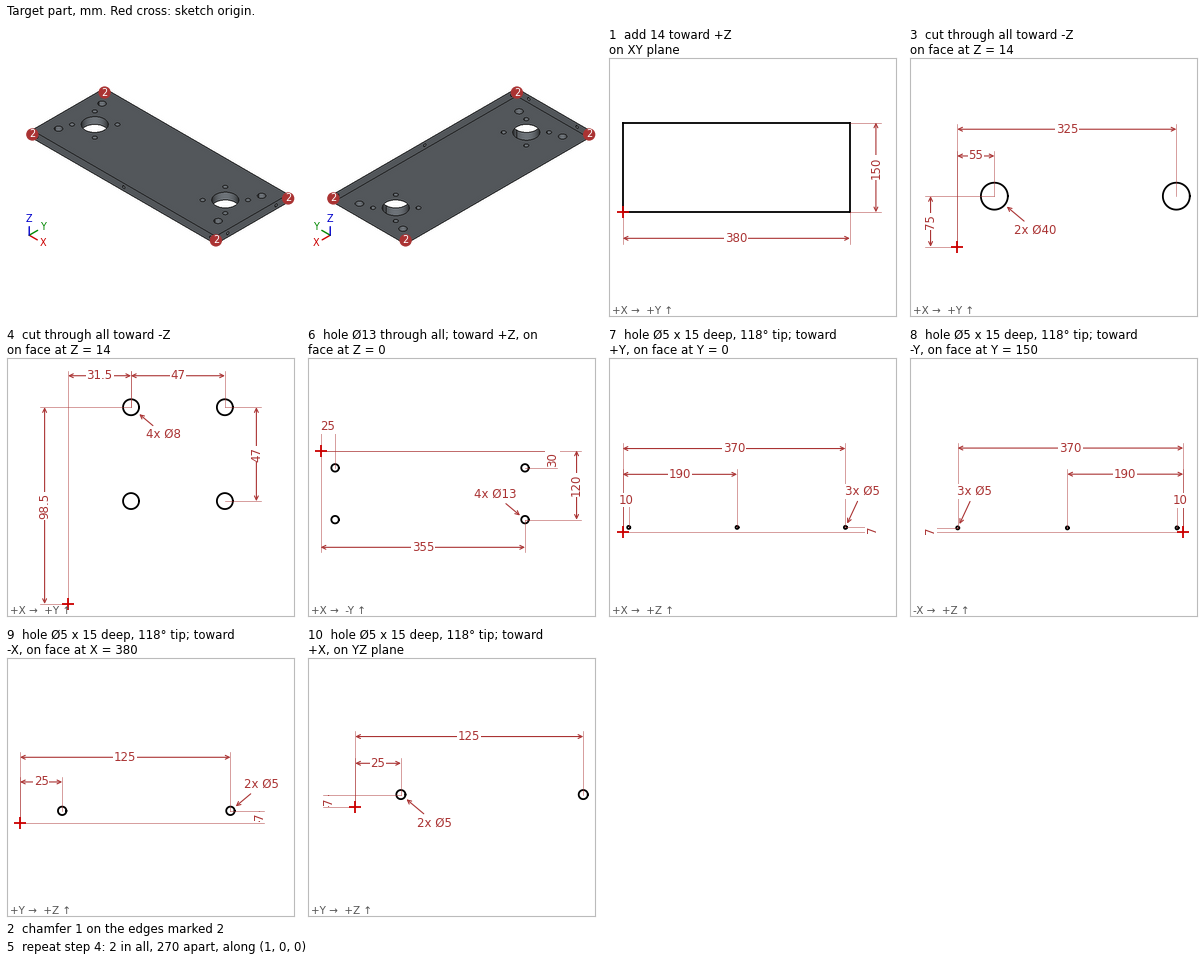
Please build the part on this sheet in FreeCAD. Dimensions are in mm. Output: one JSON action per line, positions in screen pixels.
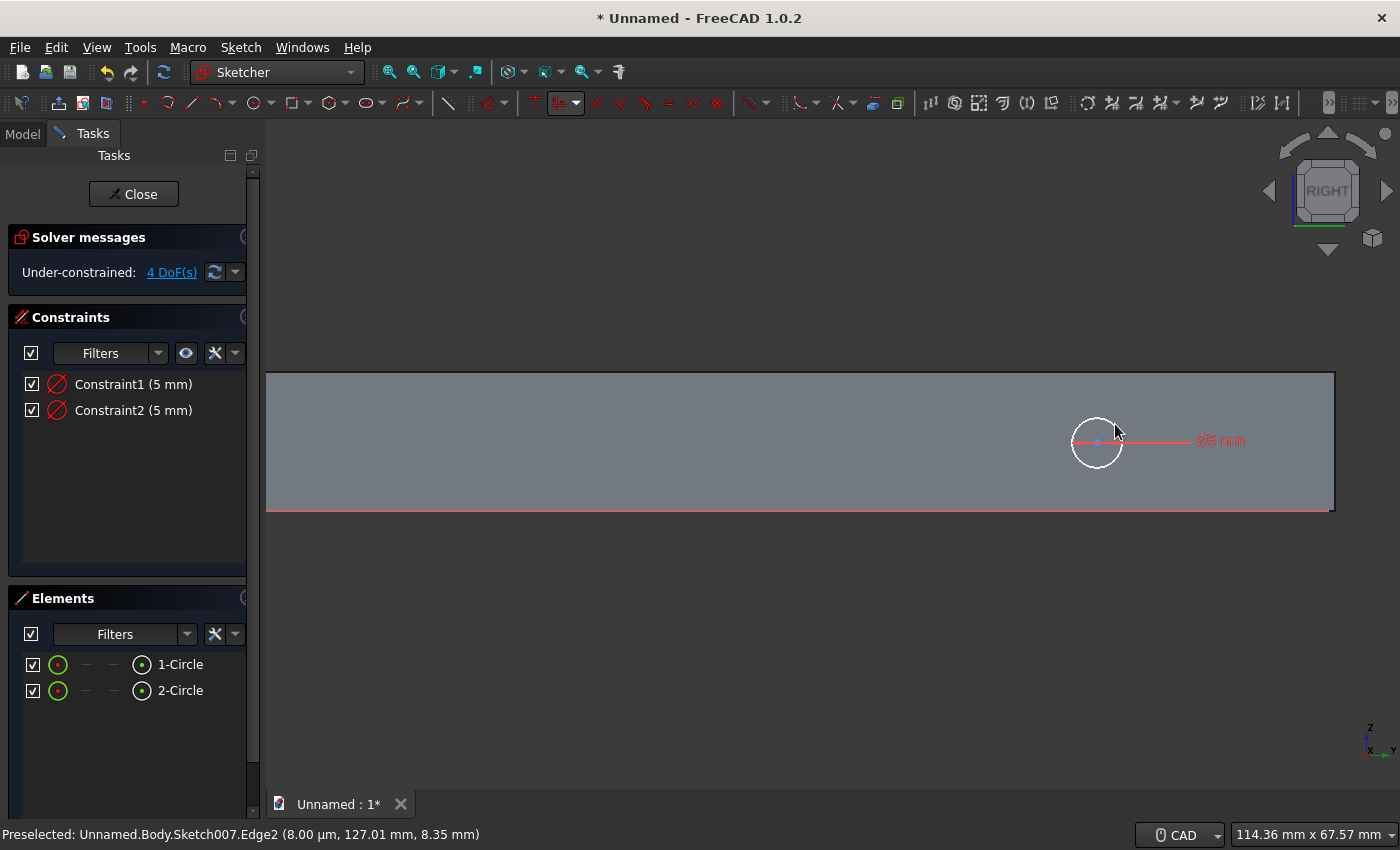
{"action": "scroll", "coordinate": [1099, 442], "scroll_direction": "down", "scroll_amount": 3}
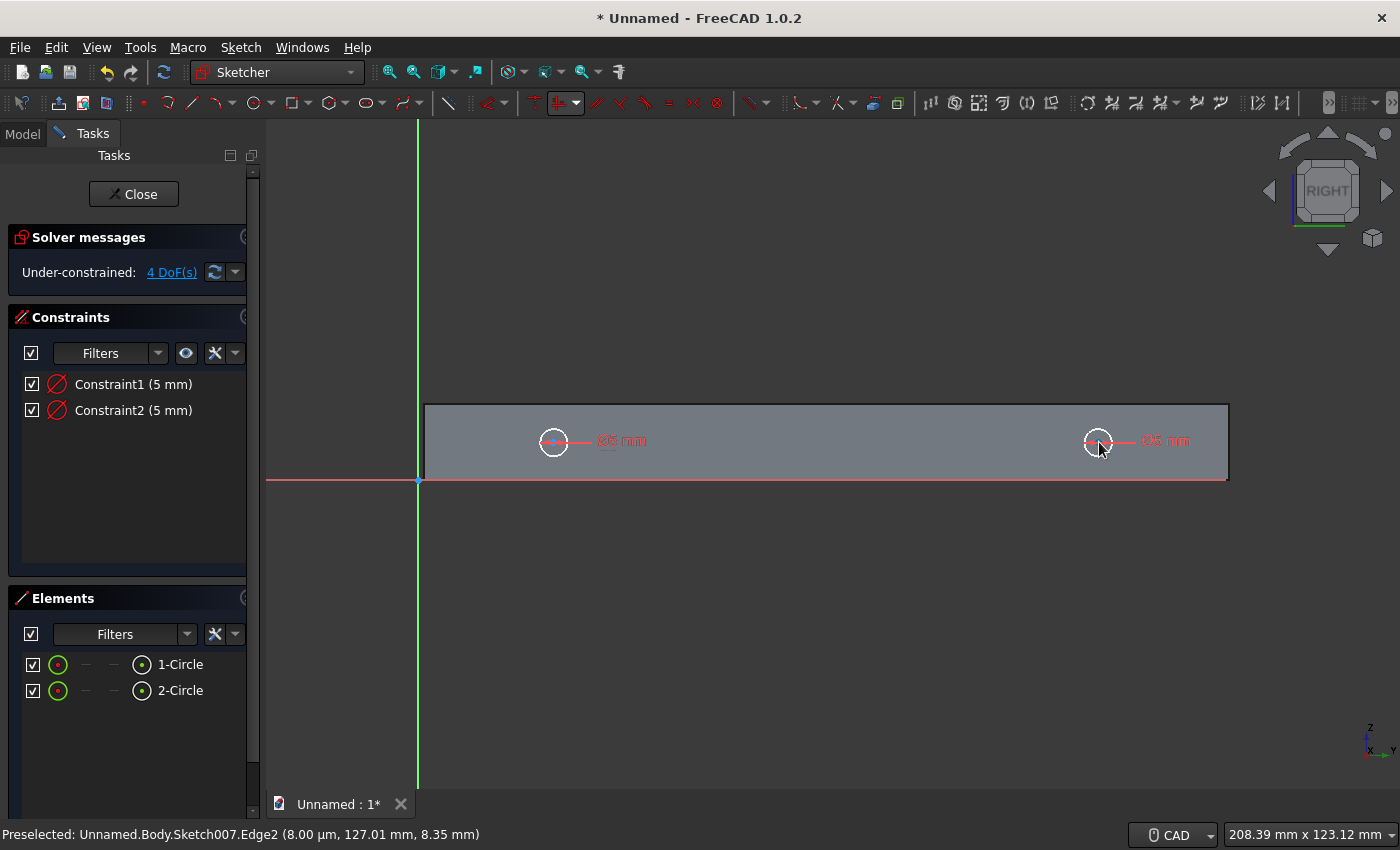
{"action": "left_click", "coordinate": [554, 443]}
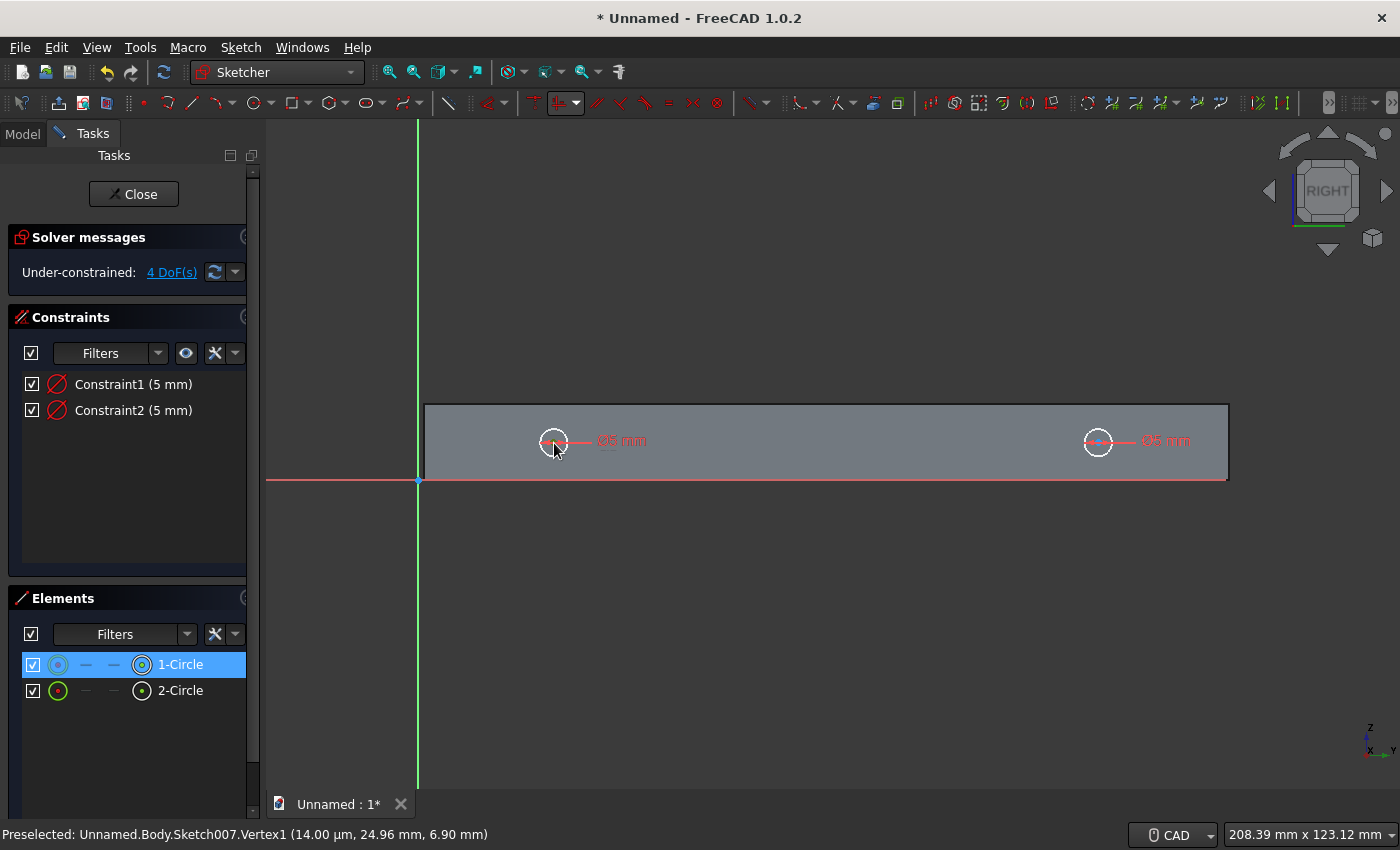
{"action": "left_click", "coordinate": [1098, 443]}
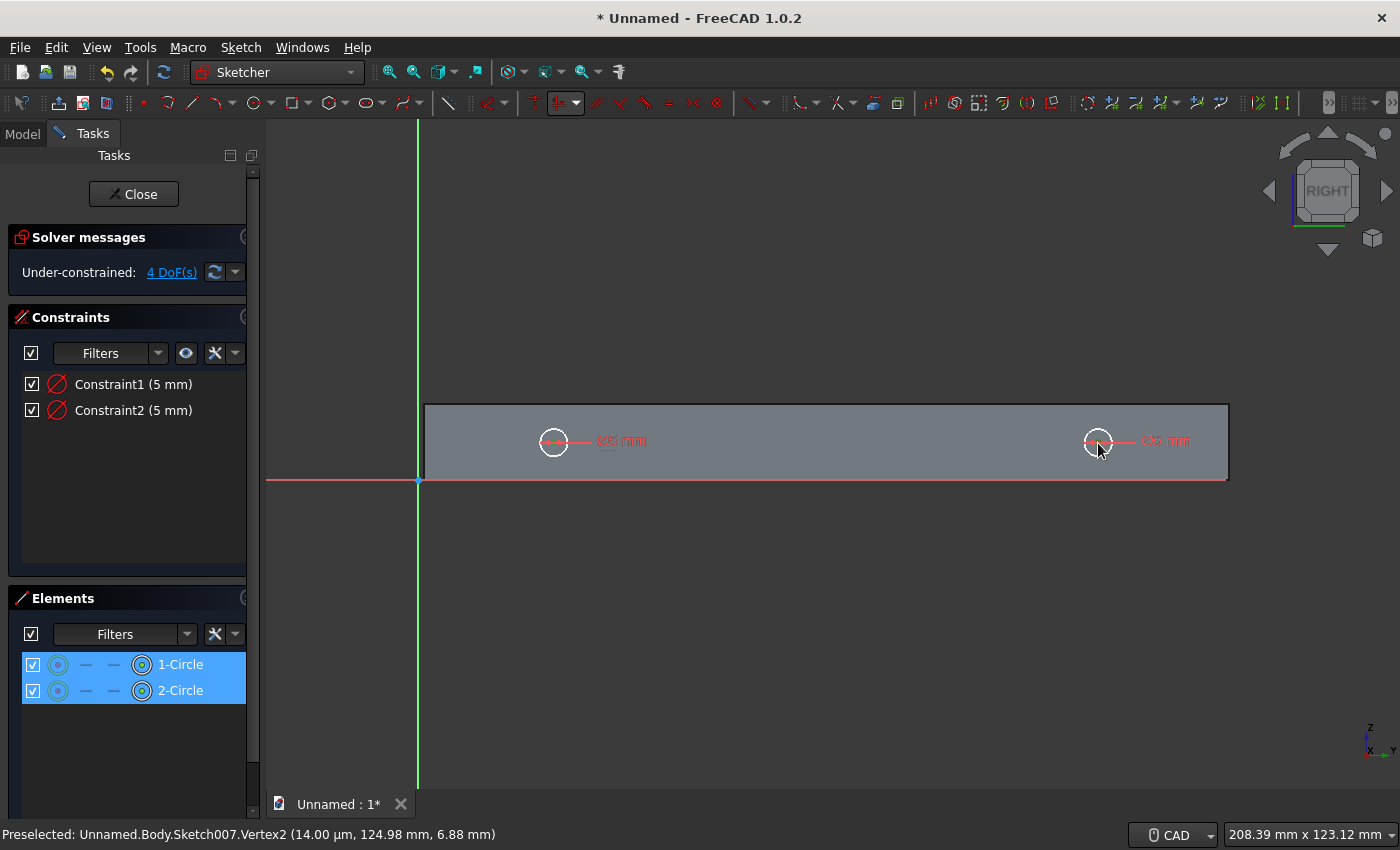
{"action": "key", "text": "h"}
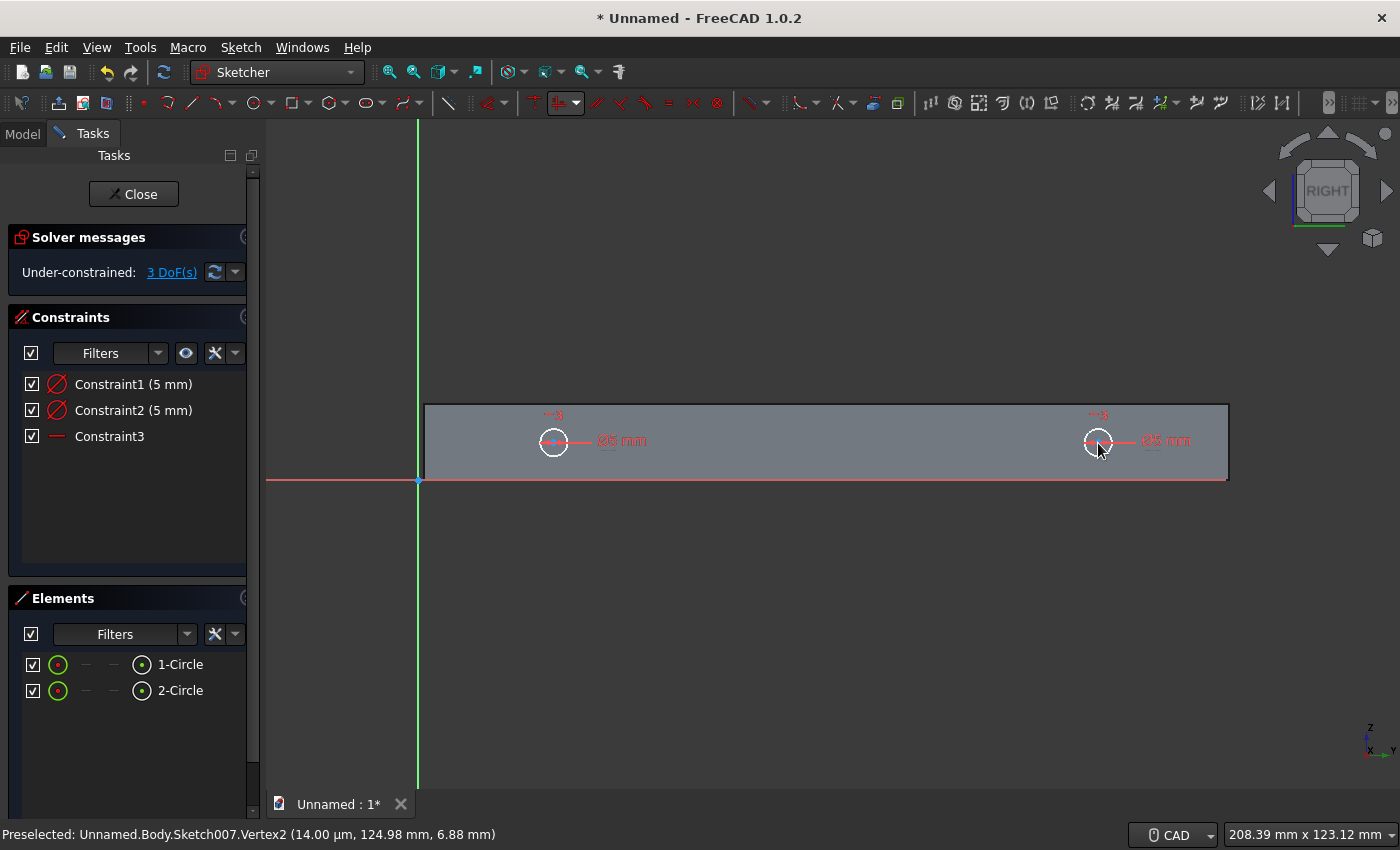
{"action": "key", "text": "d"}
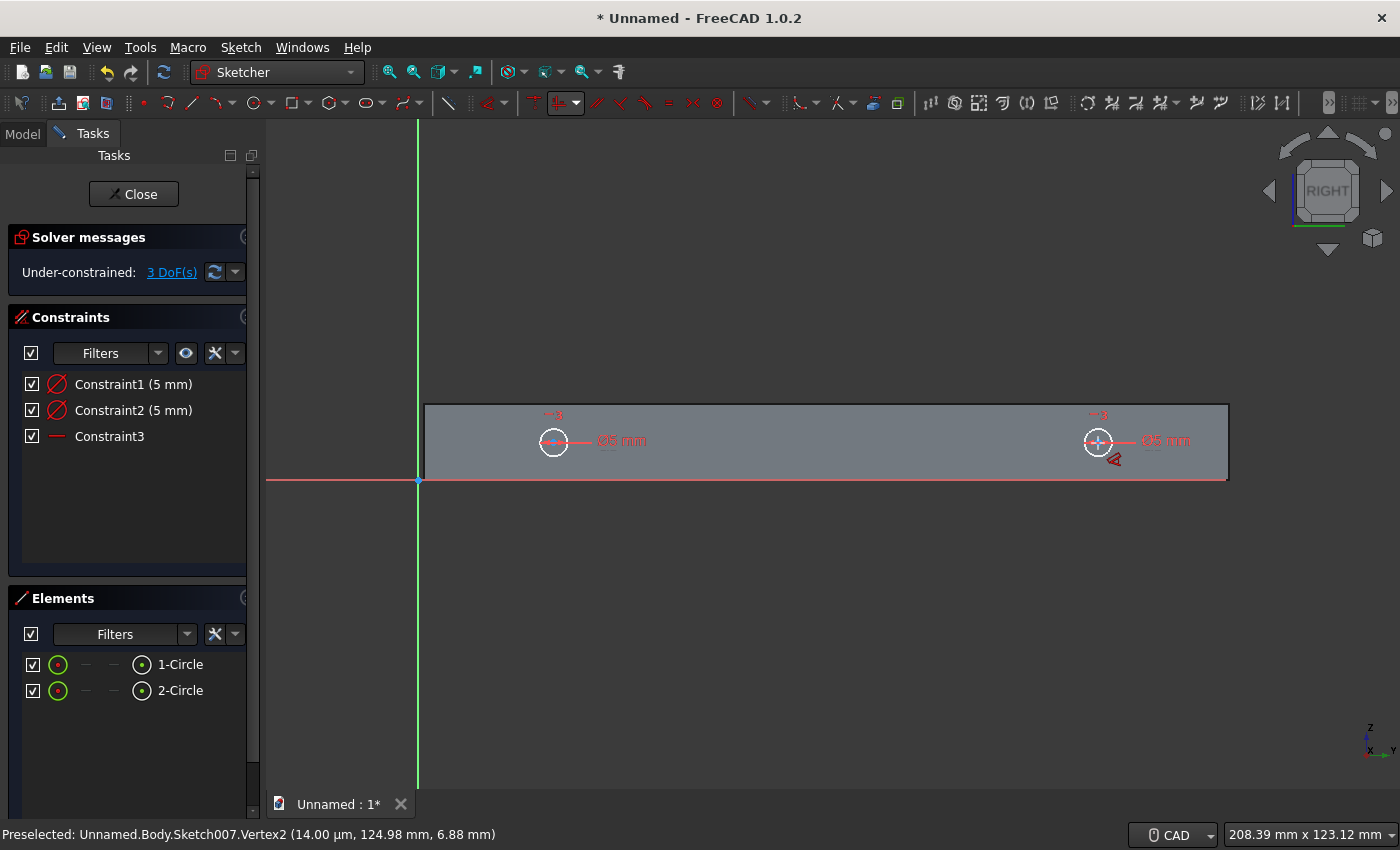
{"action": "left_click", "coordinate": [554, 443]}
{"action": "left_click", "coordinate": [384, 461]}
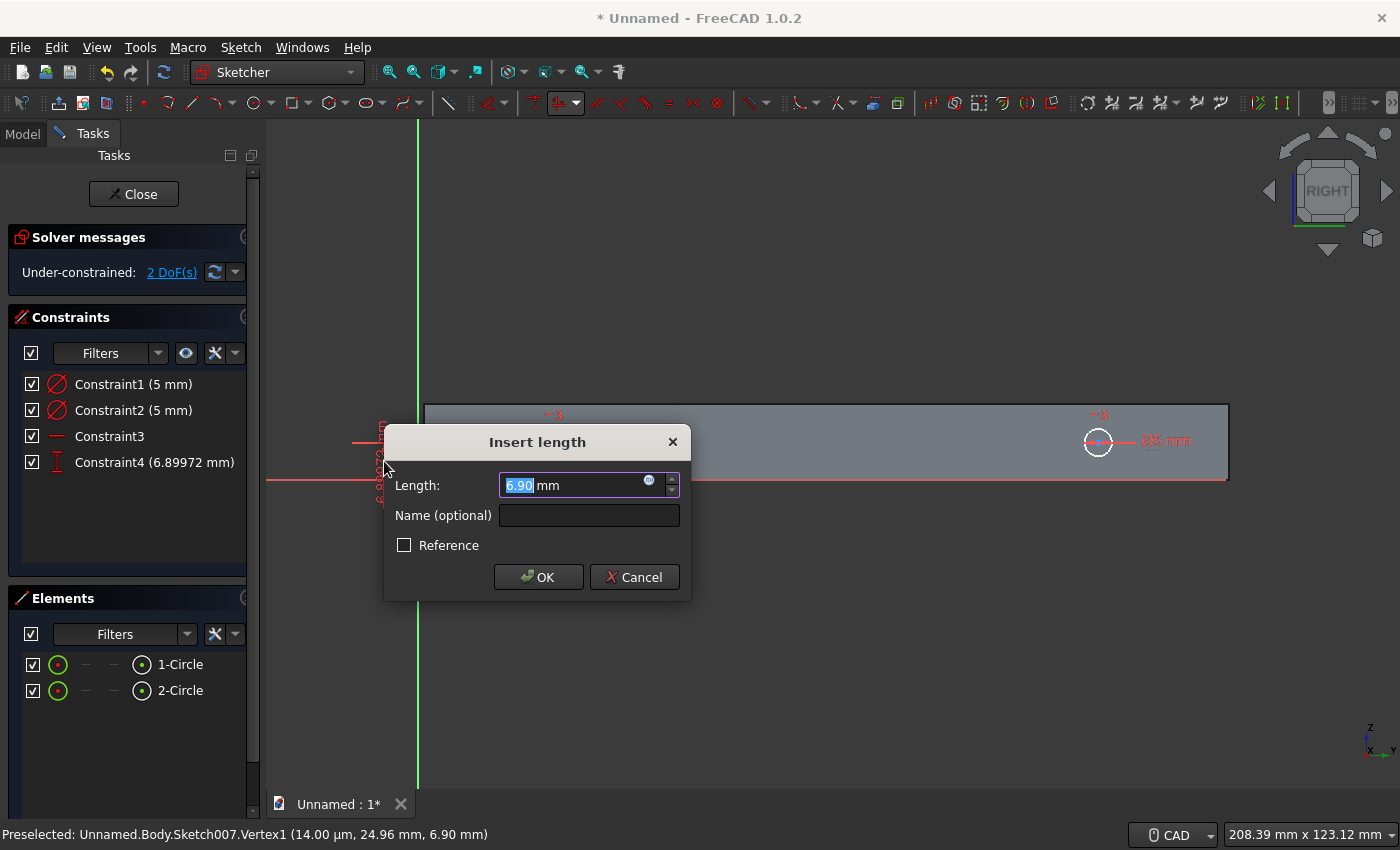
{"action": "type", "text": "7"}
{"action": "key", "text": "Return"}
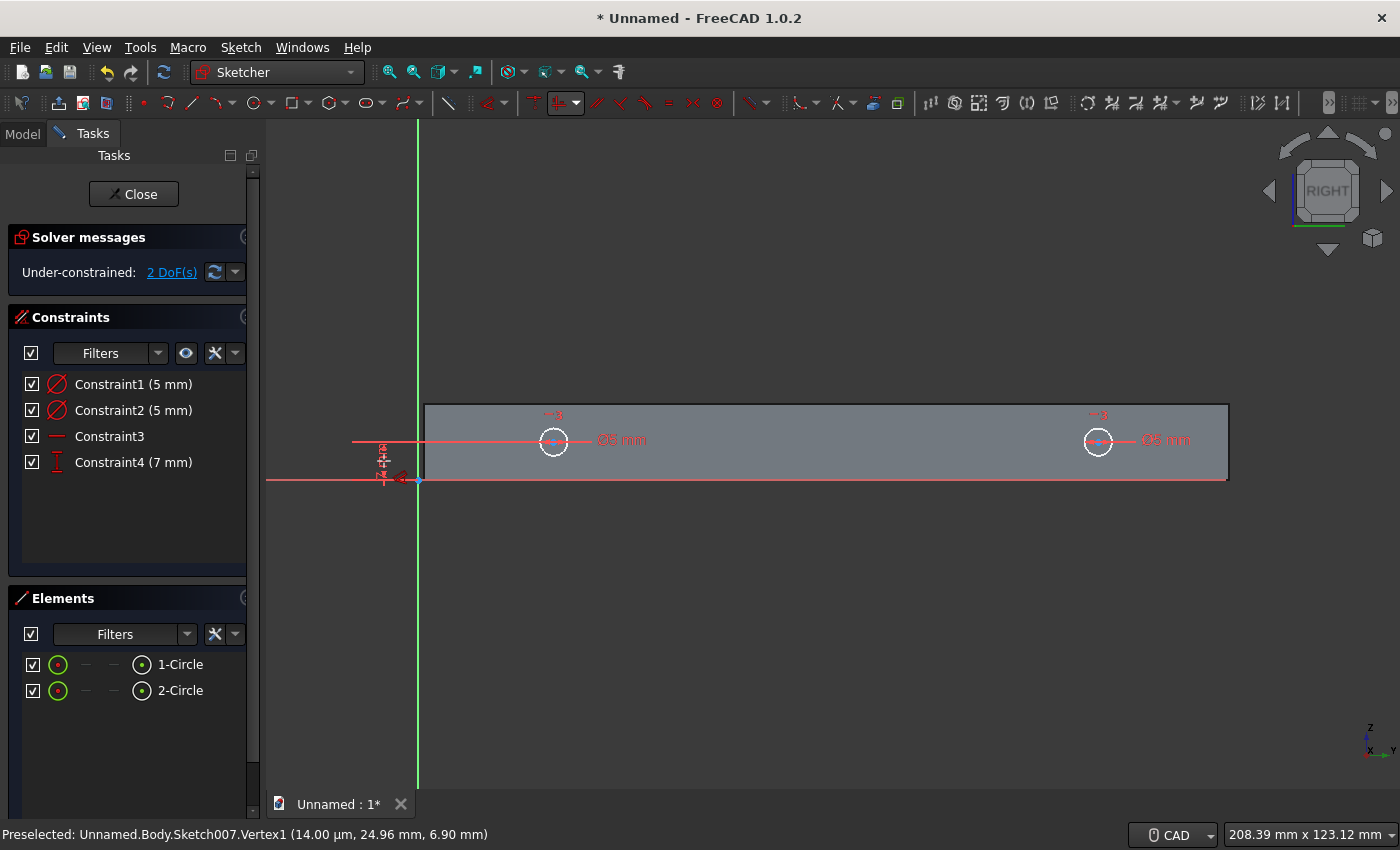
{"action": "left_click", "coordinate": [554, 442]}
{"action": "left_click", "coordinate": [486, 514]}